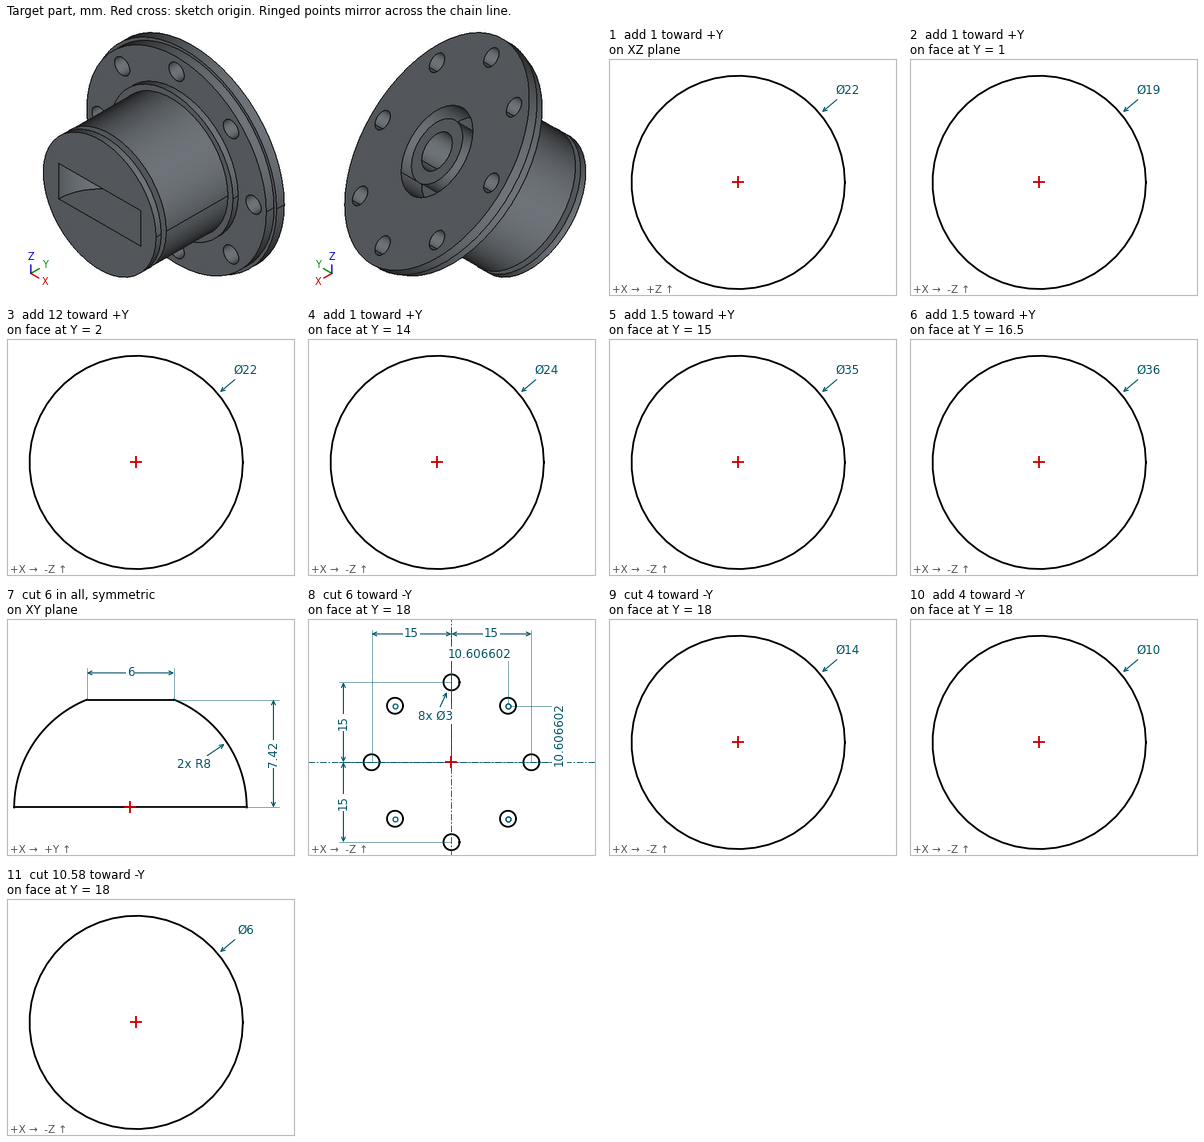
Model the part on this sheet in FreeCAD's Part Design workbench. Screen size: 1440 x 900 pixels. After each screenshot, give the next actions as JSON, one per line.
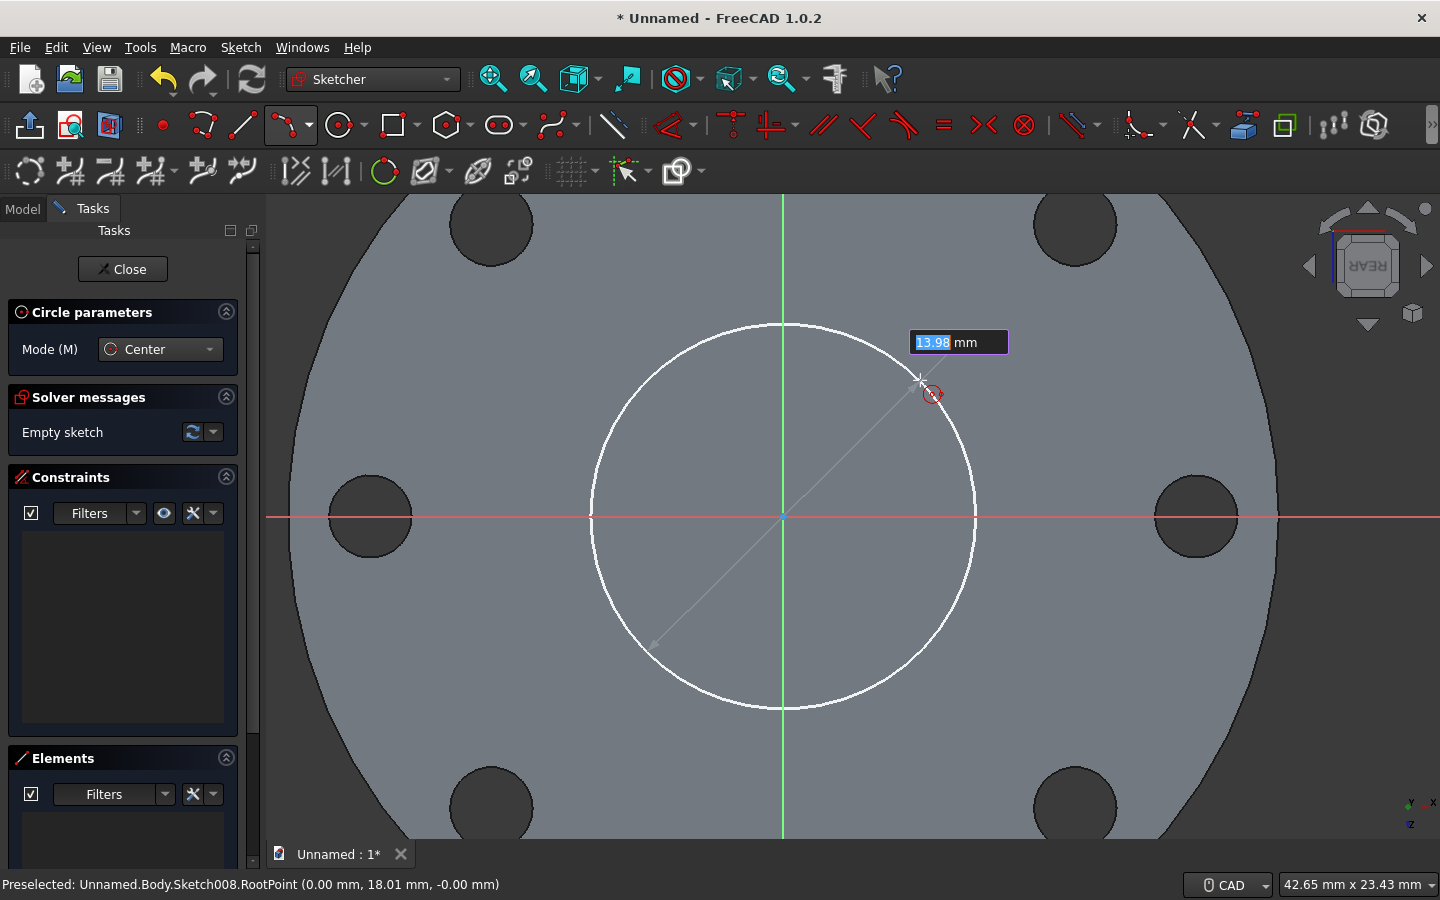
{"action": "type", "text": "14"}
{"action": "key", "text": "Return"}
{"action": "key", "text": "Escape"}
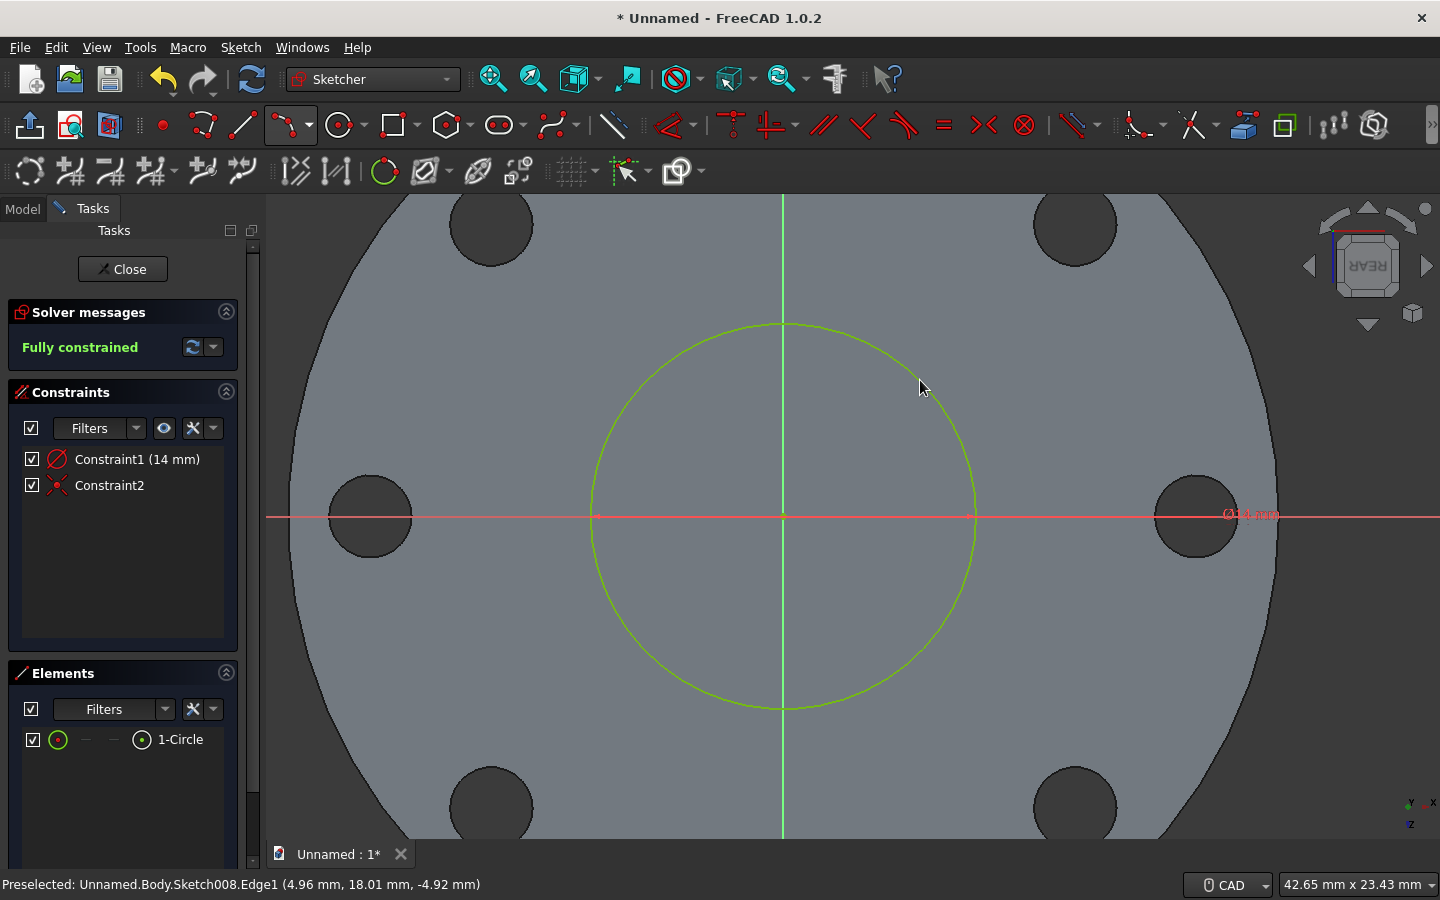
{"action": "left_click", "coordinate": [123, 269]}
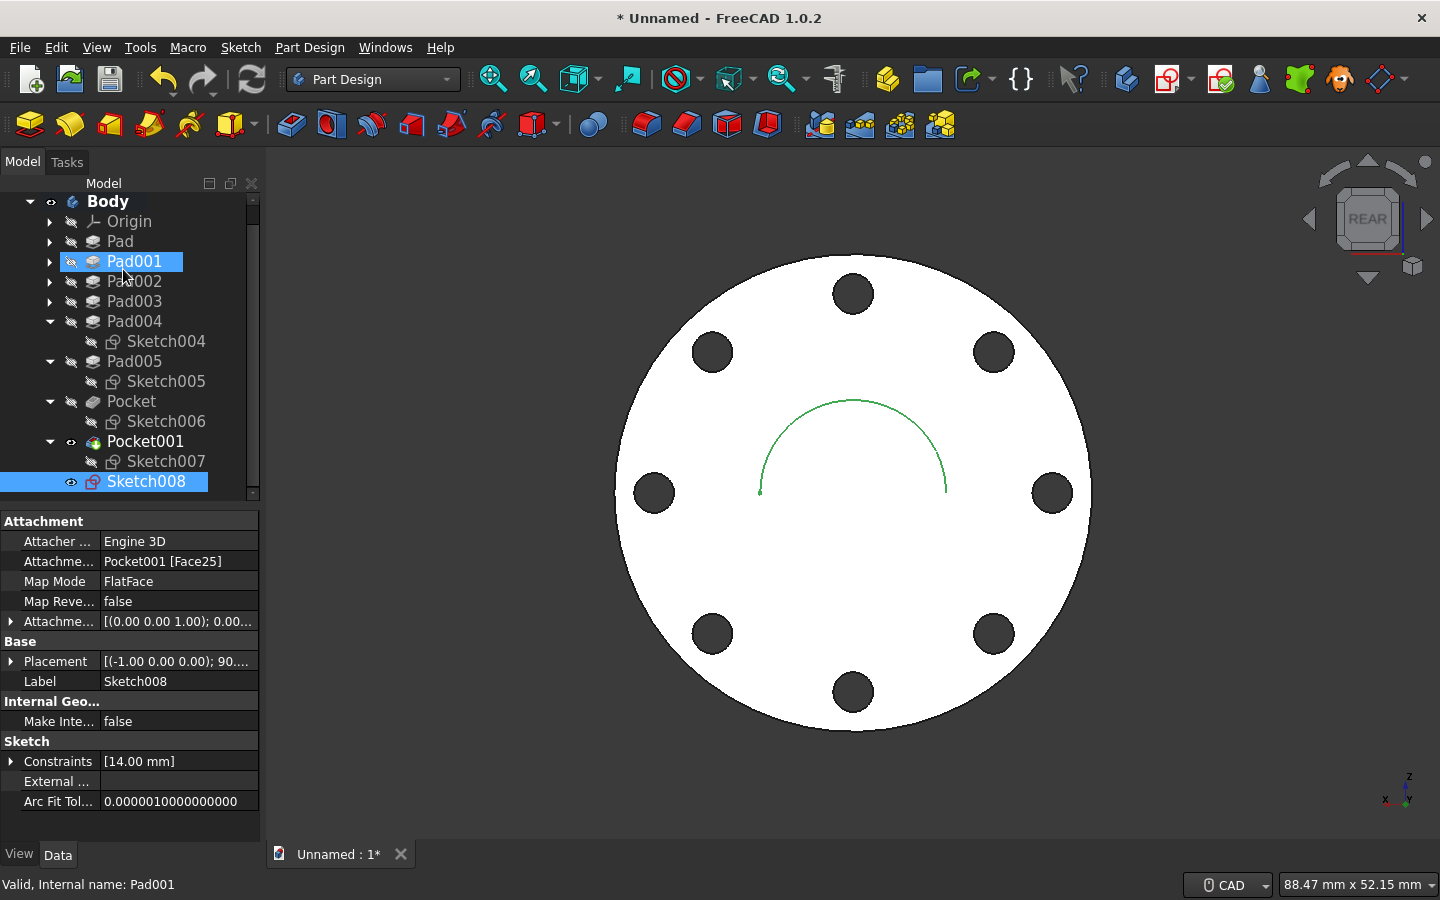
{"action": "left_click", "coordinate": [292, 124]}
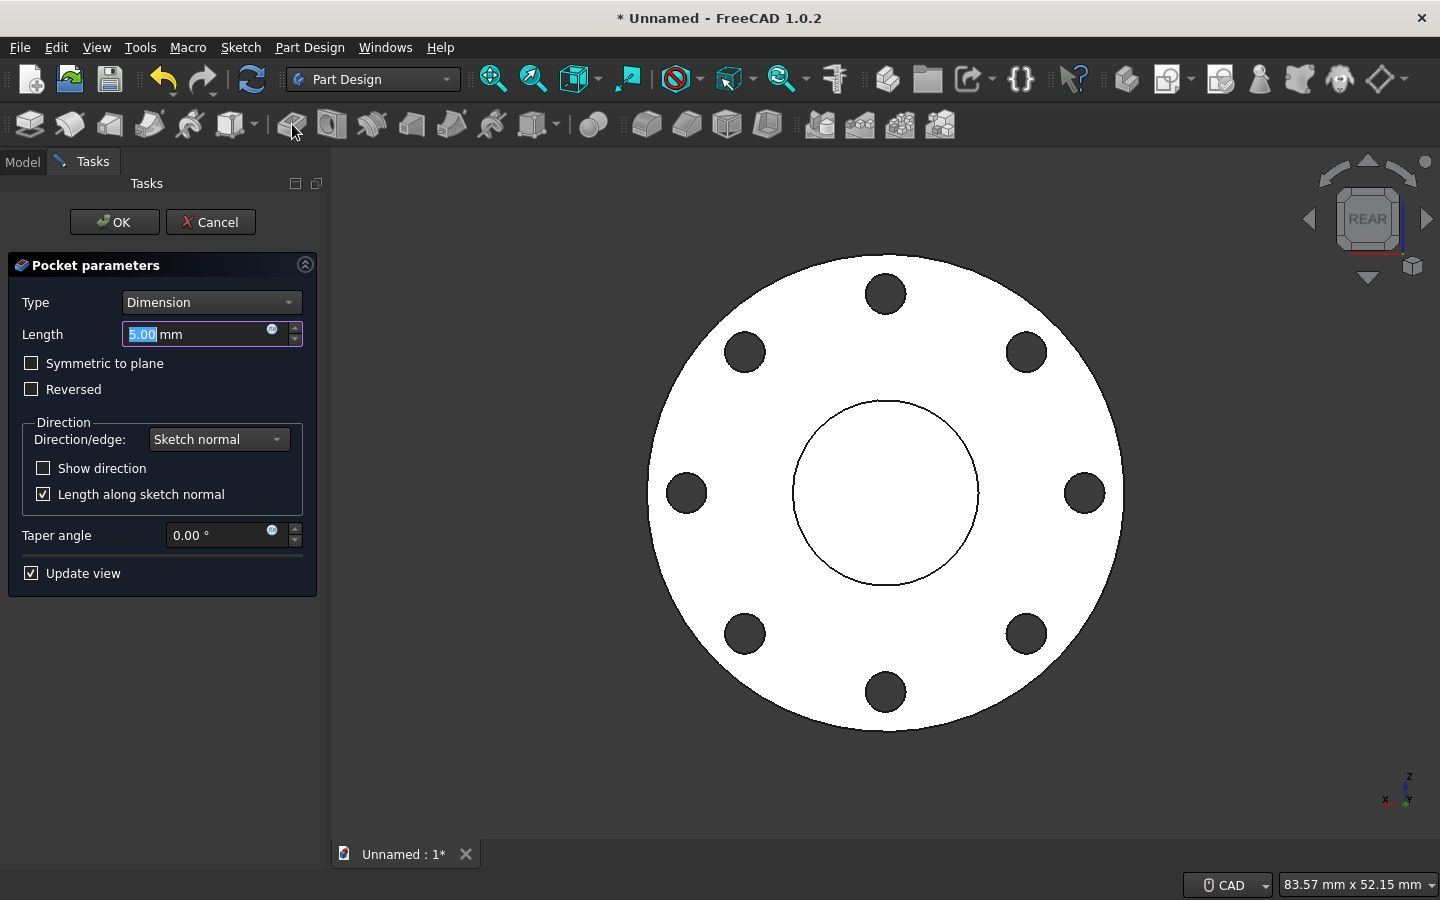
{"action": "type", "text": "4"}
{"action": "key", "text": "Tab"}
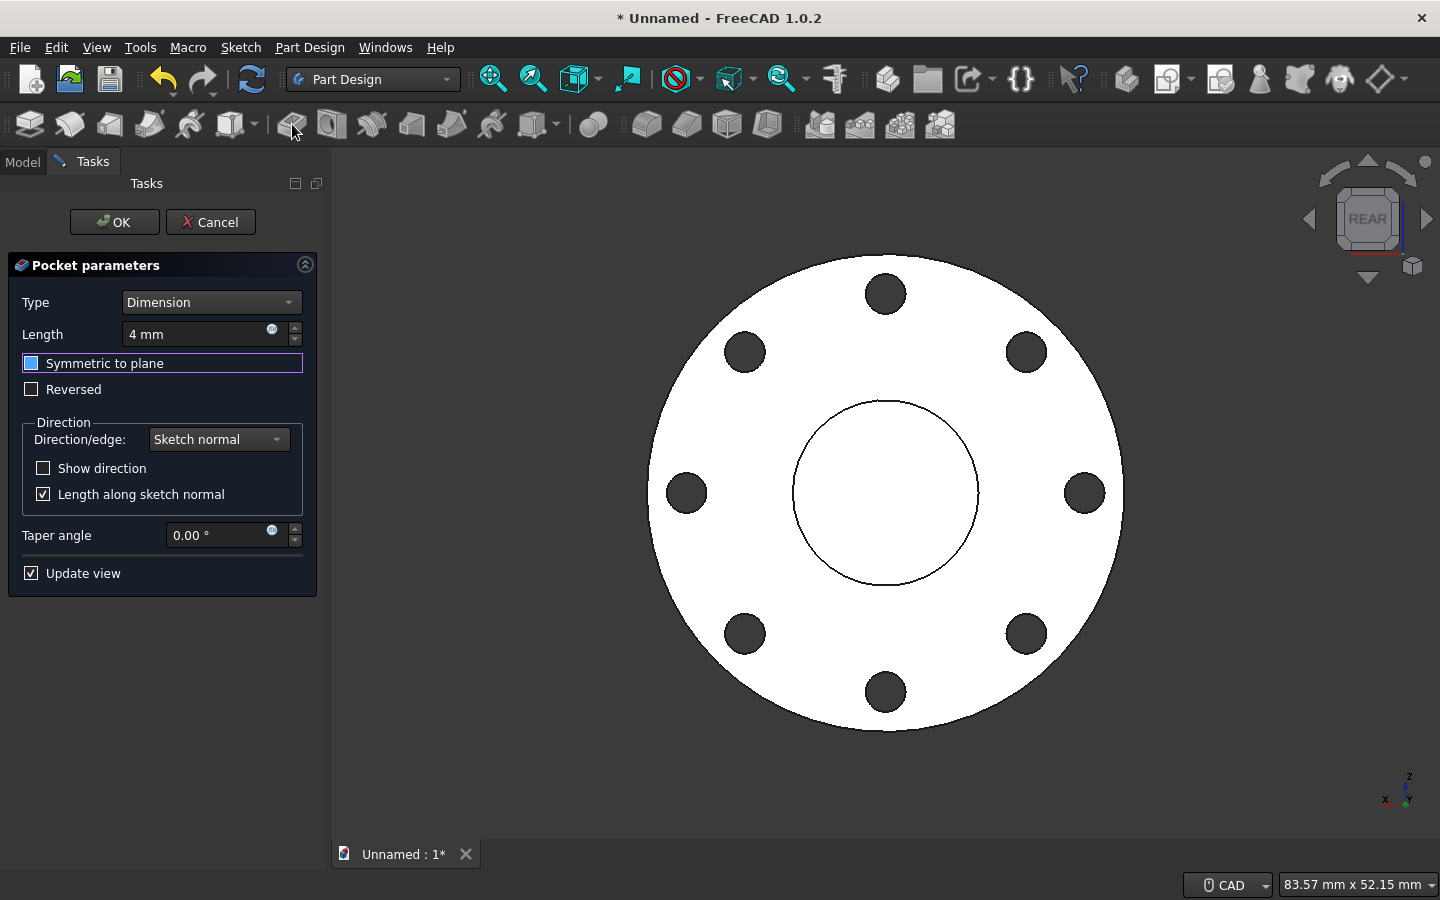
{"action": "left_click", "coordinate": [115, 222]}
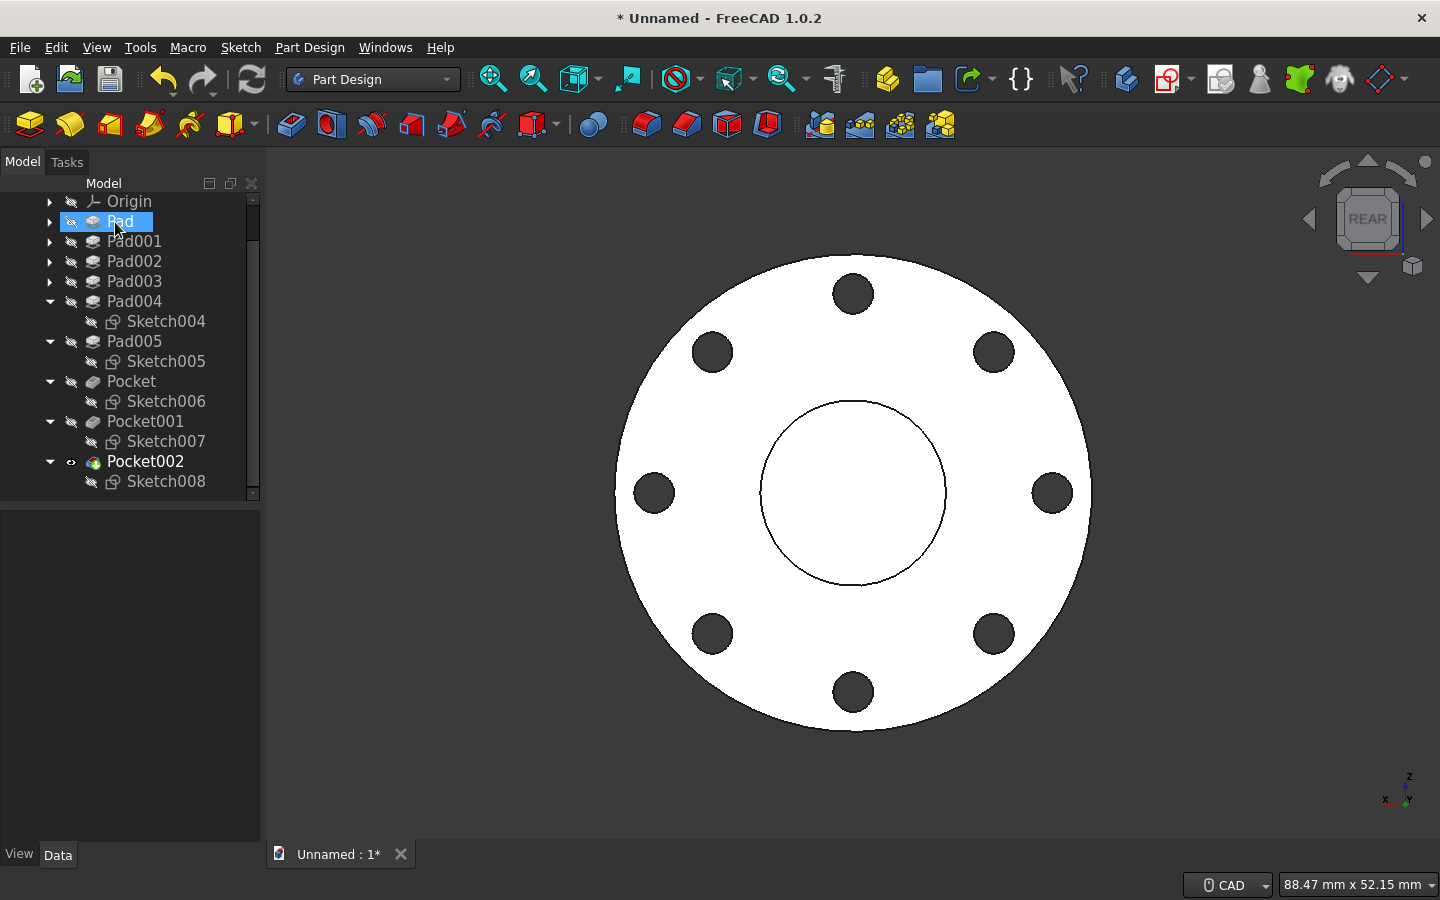
{"action": "left_click", "coordinate": [785, 628]}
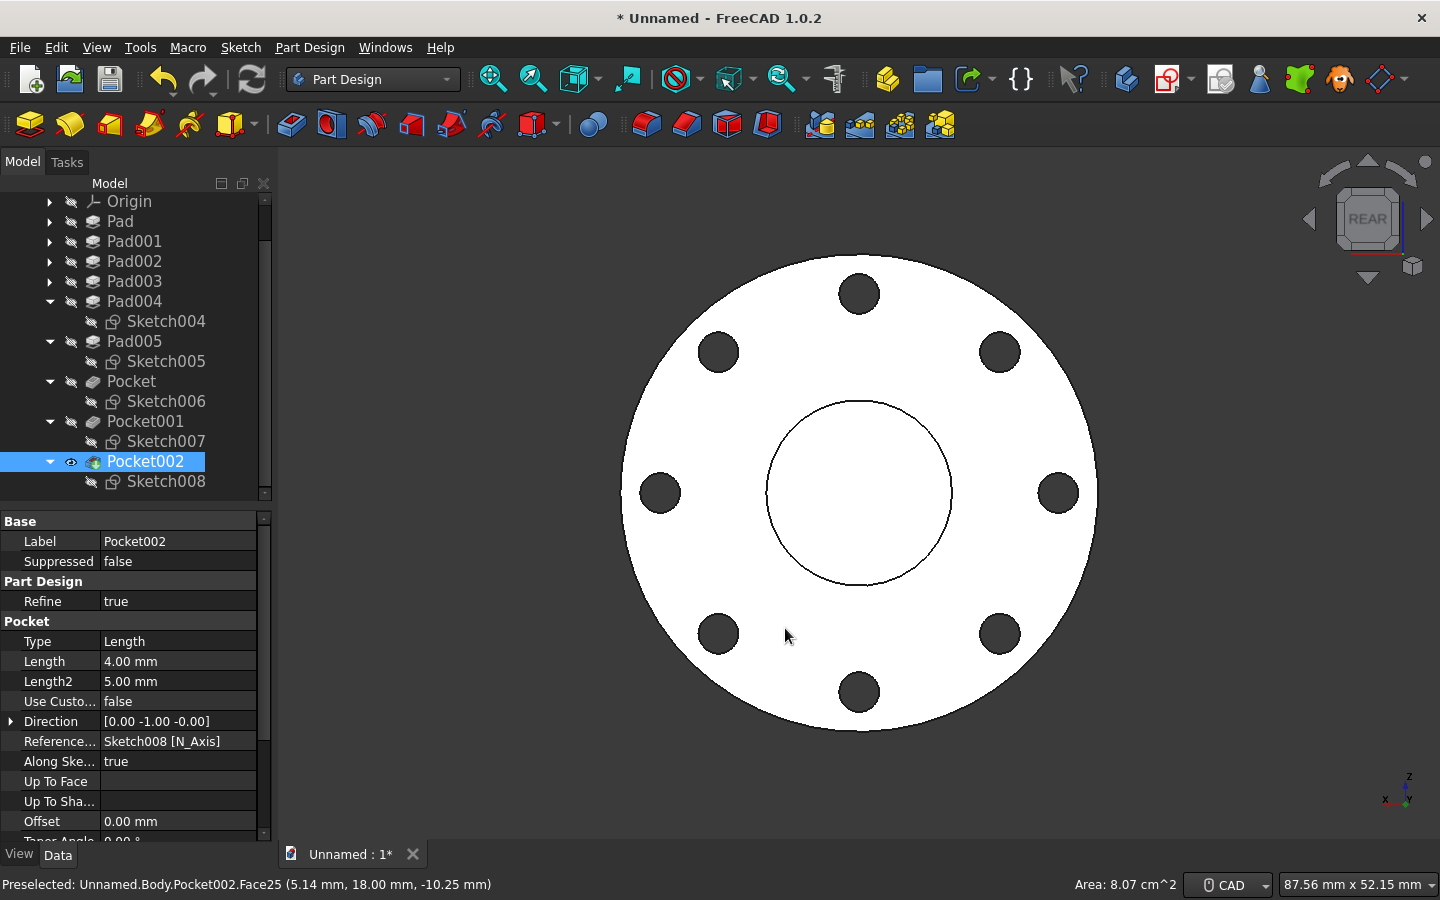
{"action": "left_click", "coordinate": [1168, 80]}